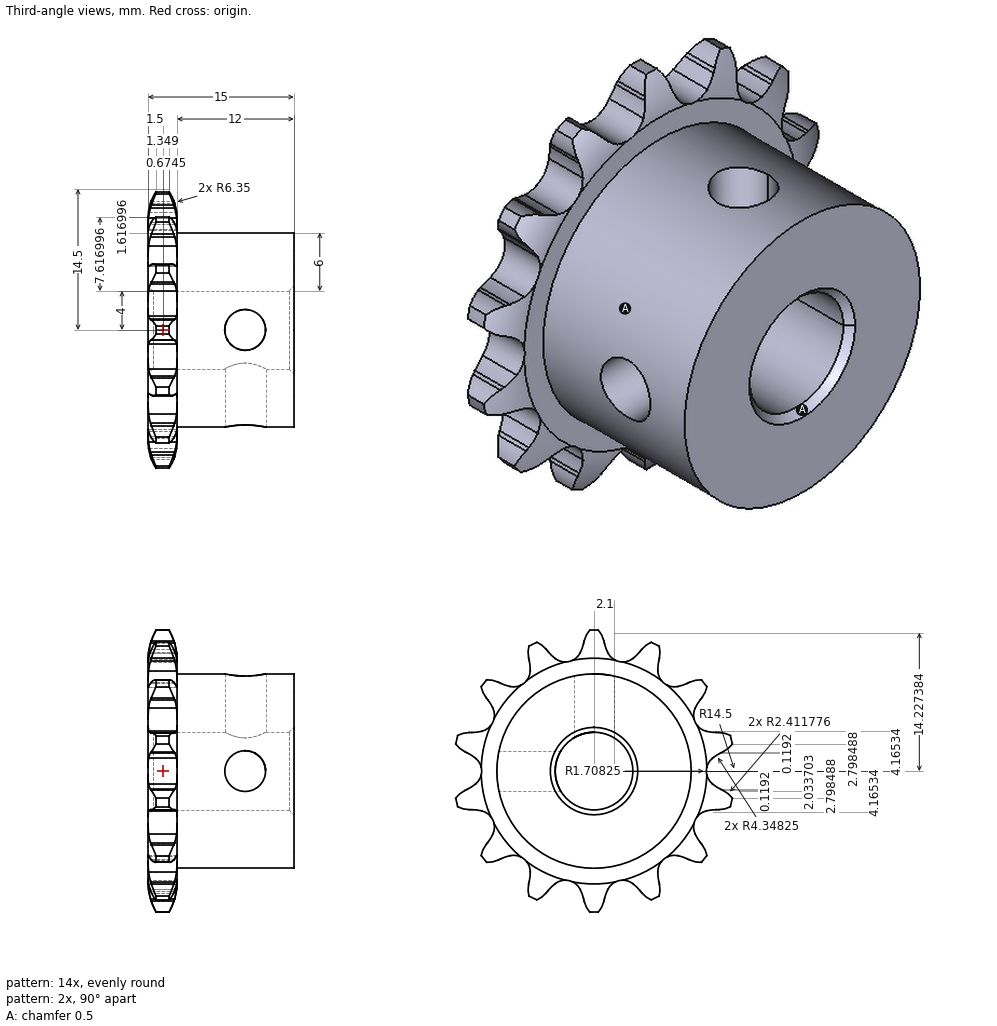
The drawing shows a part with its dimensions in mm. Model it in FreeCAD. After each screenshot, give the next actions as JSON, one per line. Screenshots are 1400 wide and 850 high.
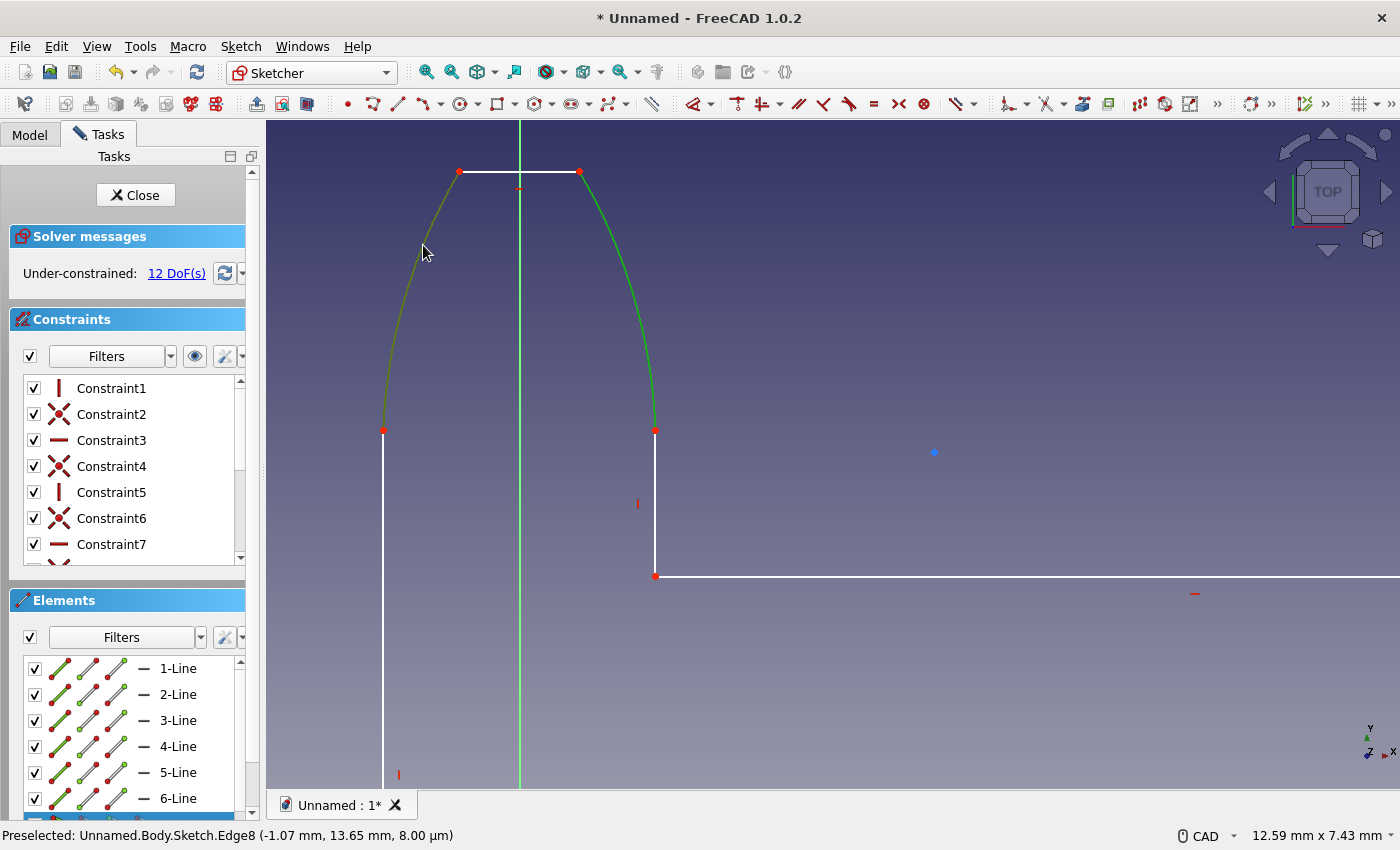
{"action": "left_click", "coordinate": [874, 104]}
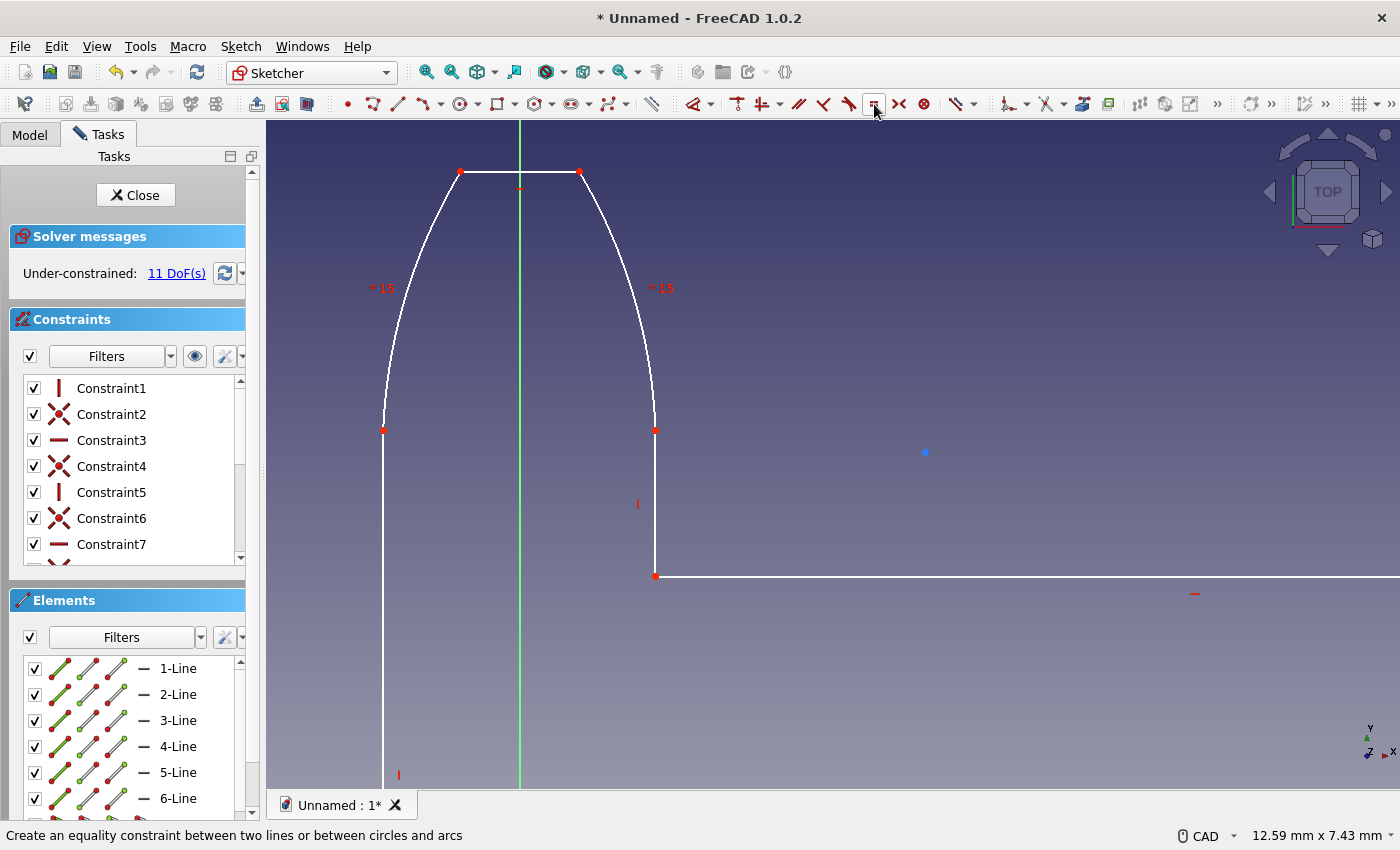
{"action": "left_click", "coordinate": [692, 104]}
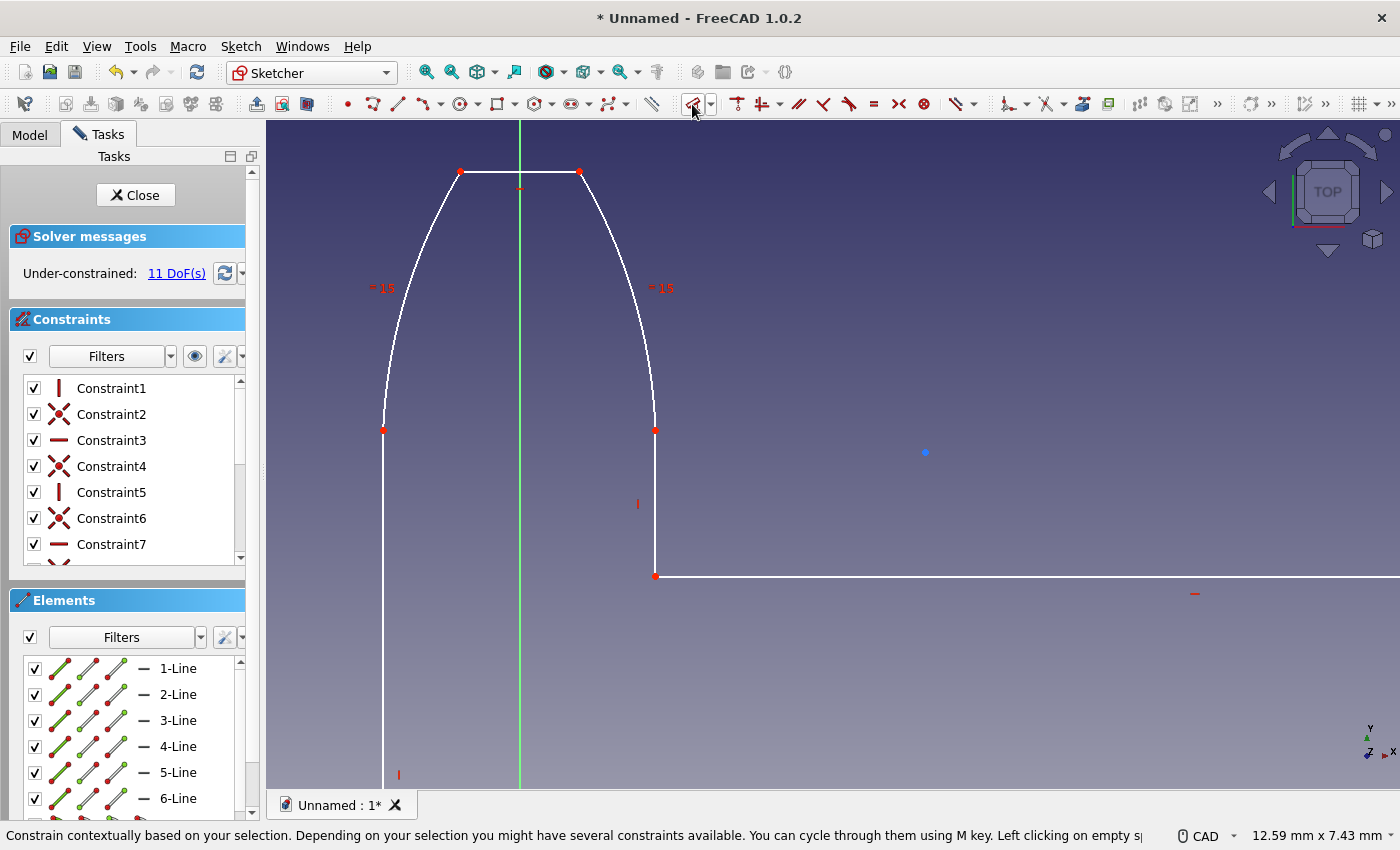
{"action": "left_click", "coordinate": [646, 349]}
{"action": "left_click", "coordinate": [677, 343]}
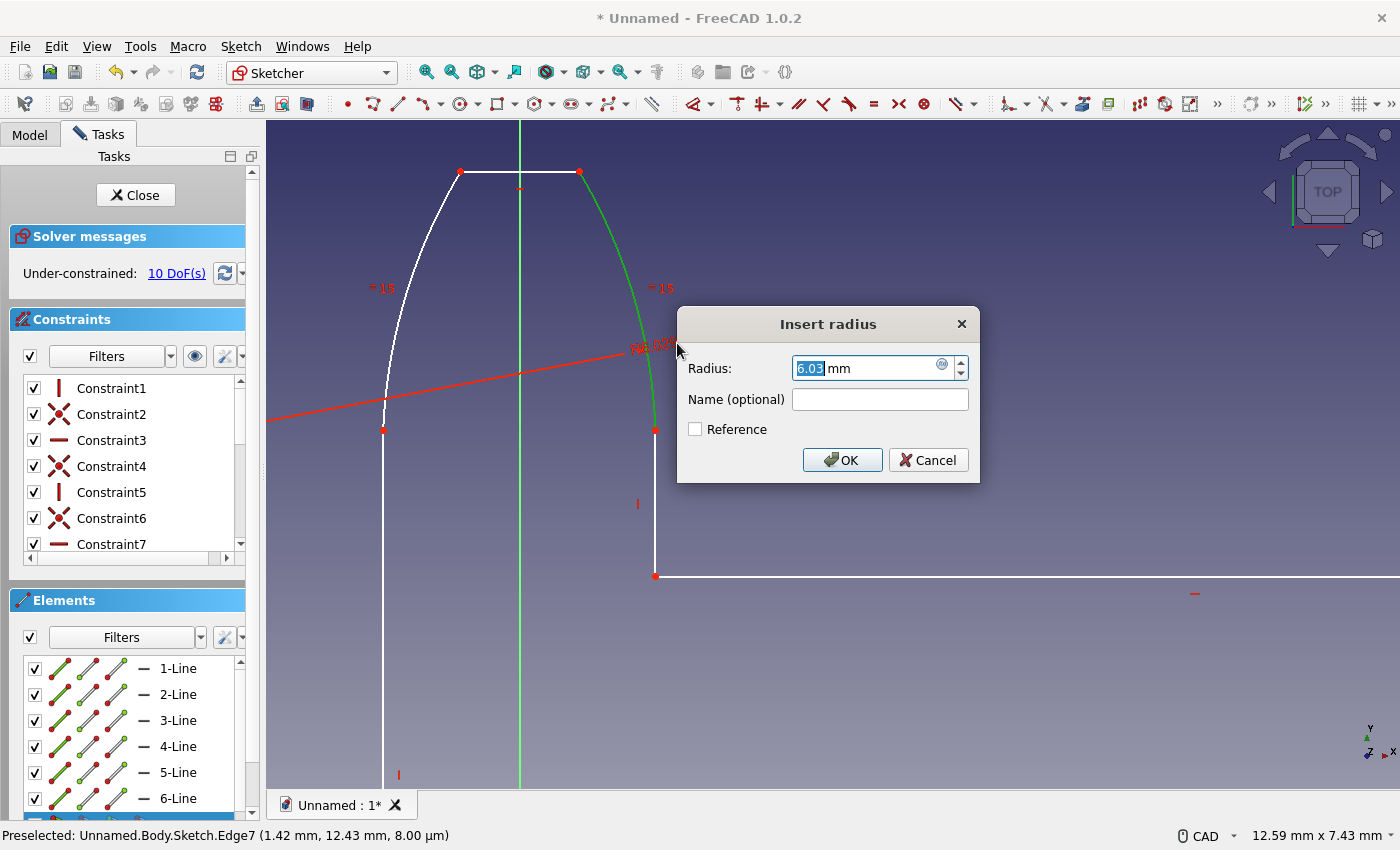
{"action": "type", "text": "6.35"}
{"action": "key", "text": "Return"}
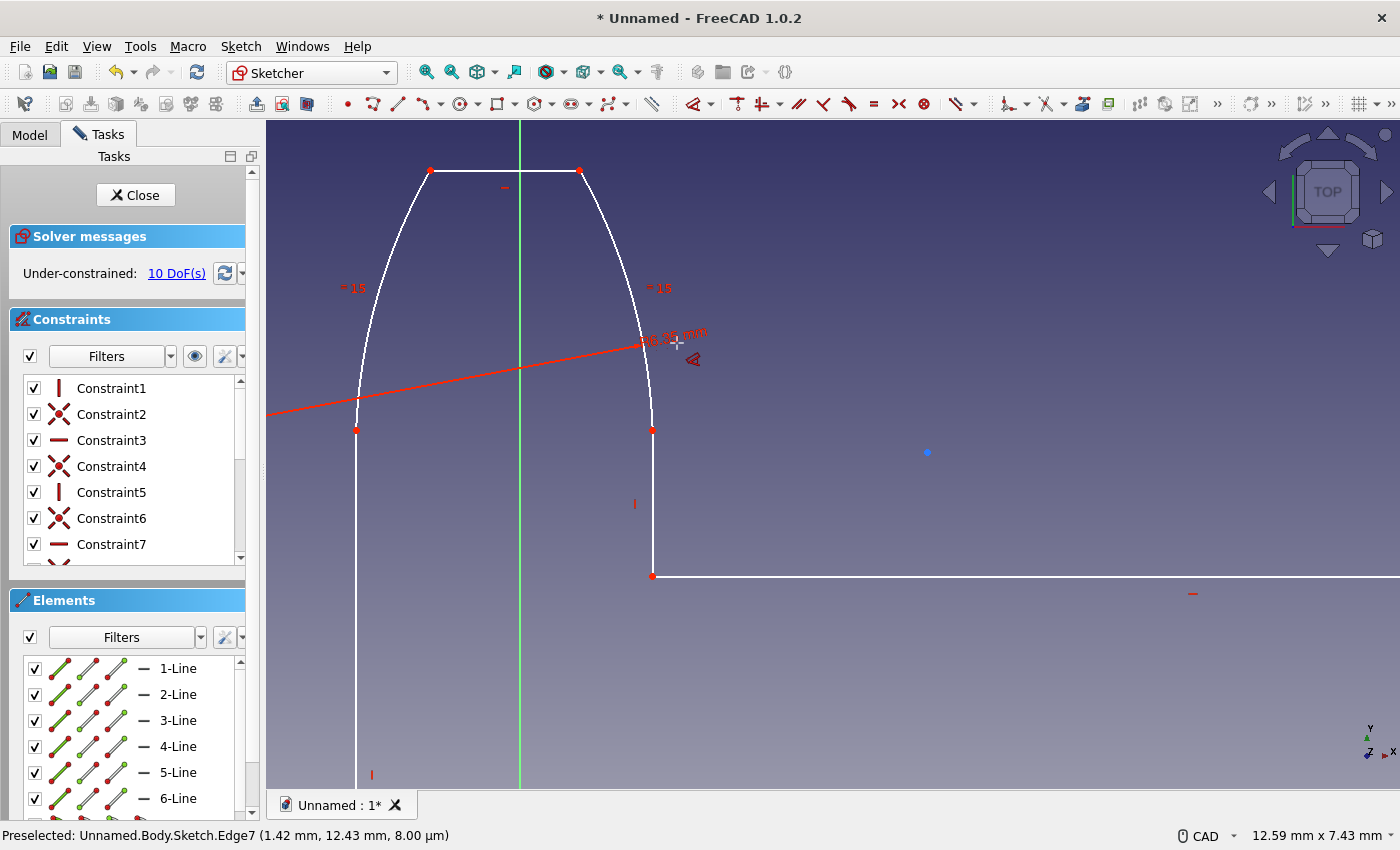
{"action": "scroll", "coordinate": [637, 296], "scroll_direction": "down", "scroll_amount": 6}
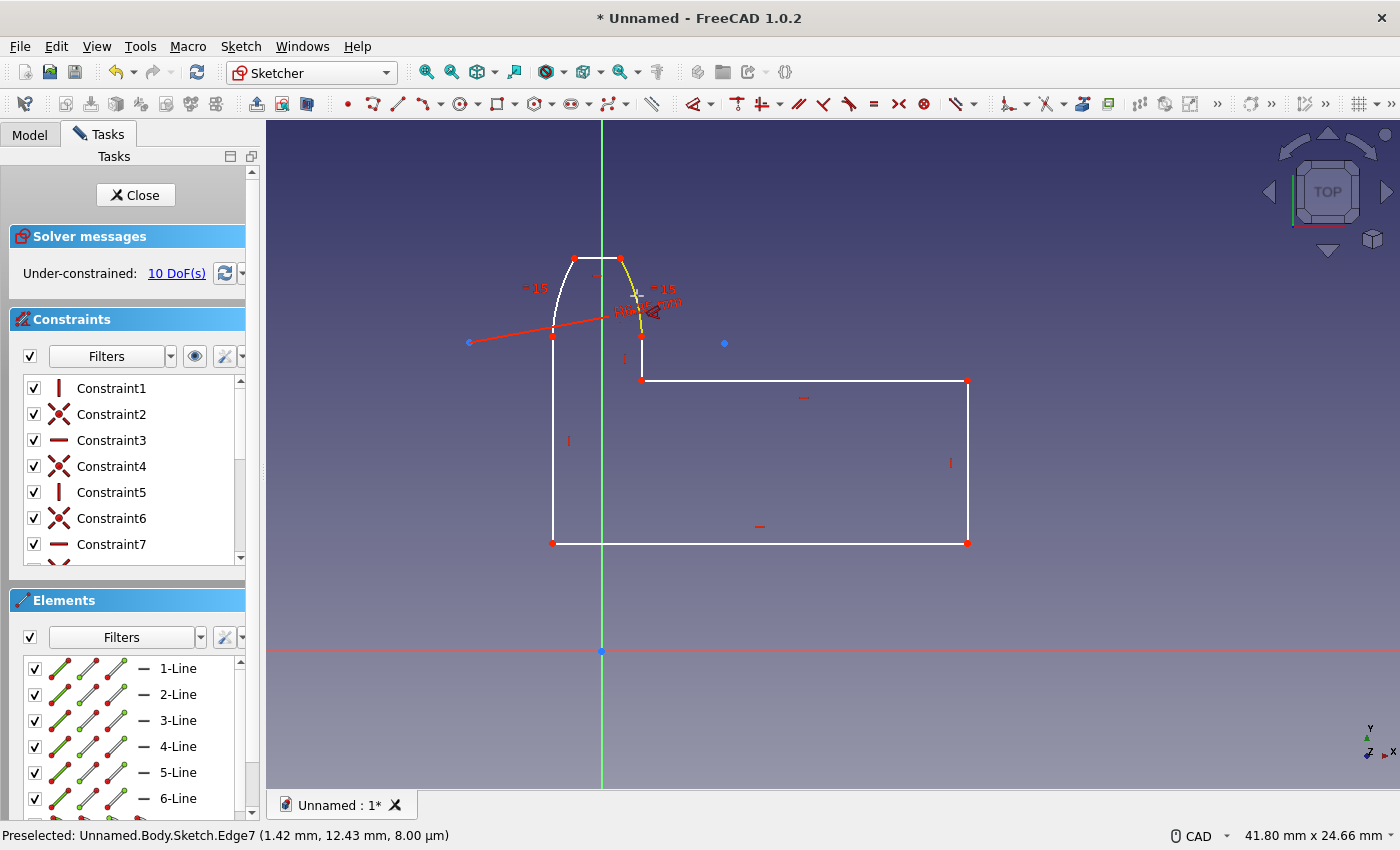
{"action": "left_click", "coordinate": [968, 495]}
{"action": "left_click", "coordinate": [1002, 462]}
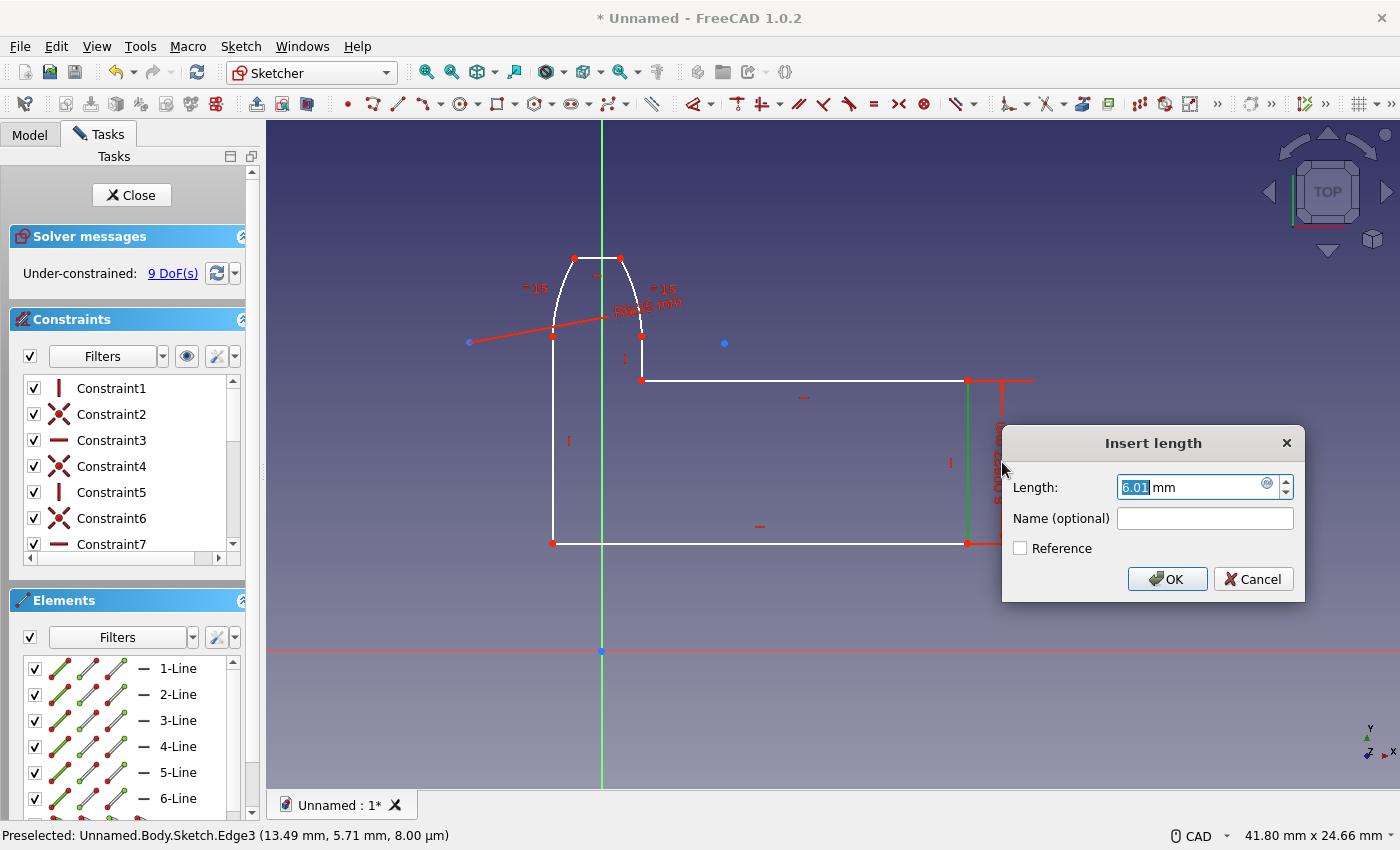
{"action": "type", "text": "6"}
{"action": "key", "text": "Return"}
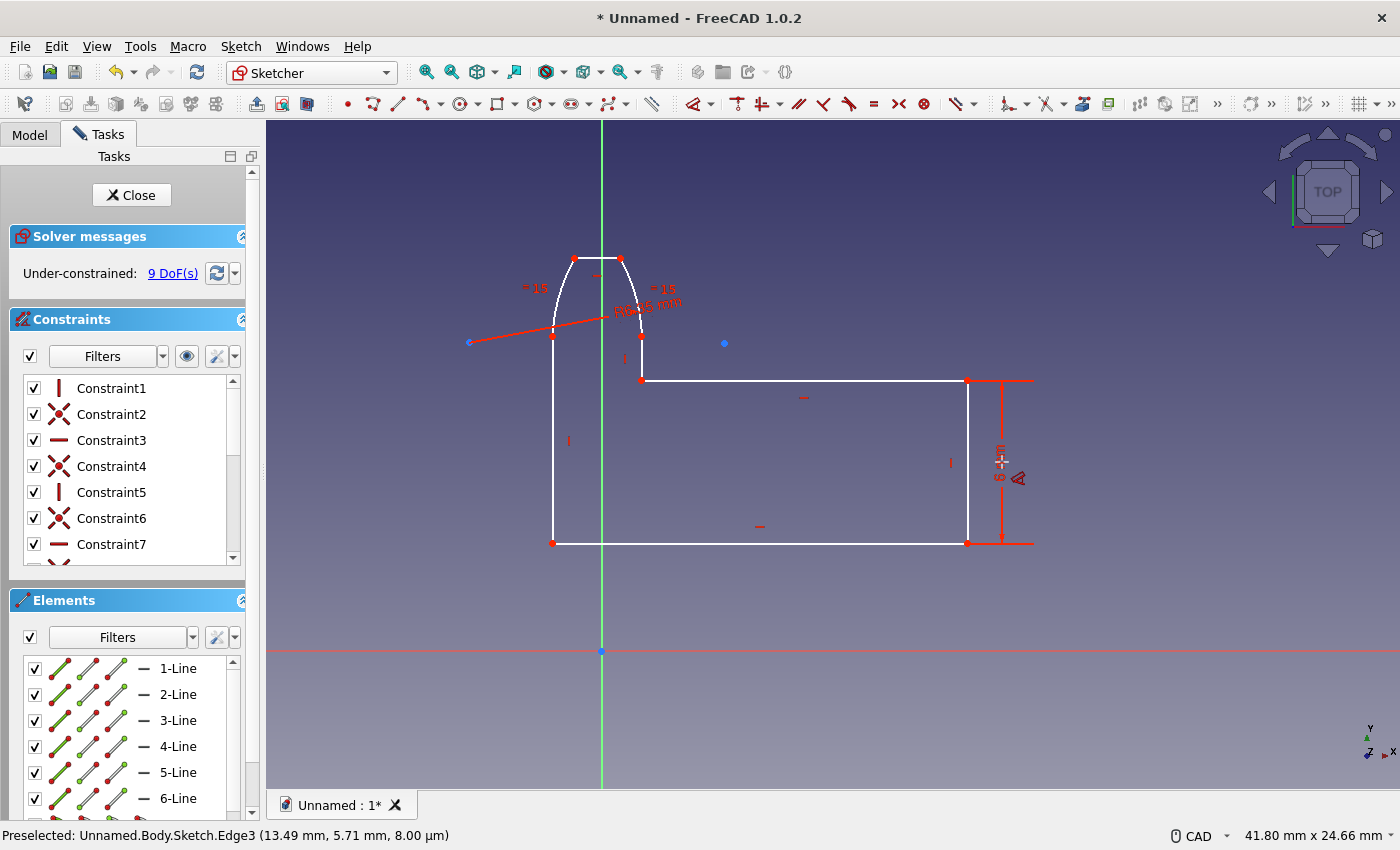
{"action": "left_click", "coordinate": [677, 544]}
{"action": "left_click", "coordinate": [760, 578]}